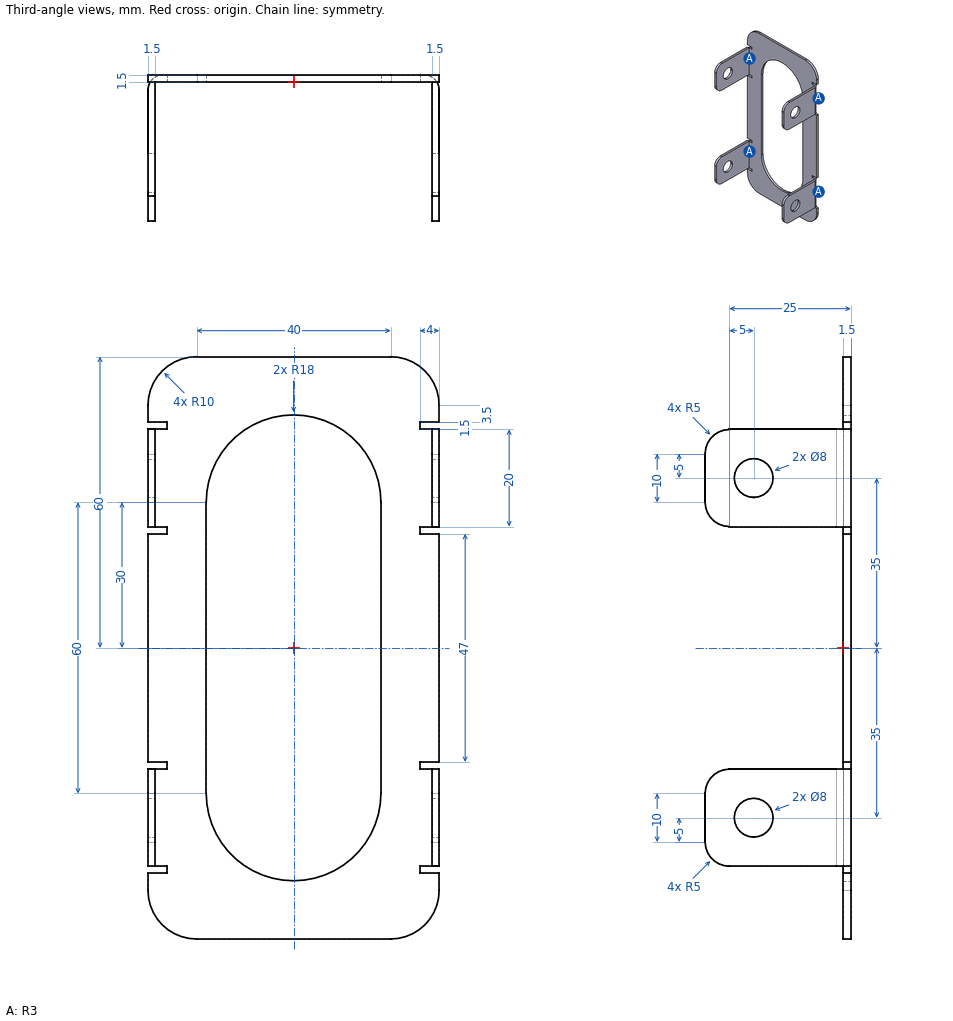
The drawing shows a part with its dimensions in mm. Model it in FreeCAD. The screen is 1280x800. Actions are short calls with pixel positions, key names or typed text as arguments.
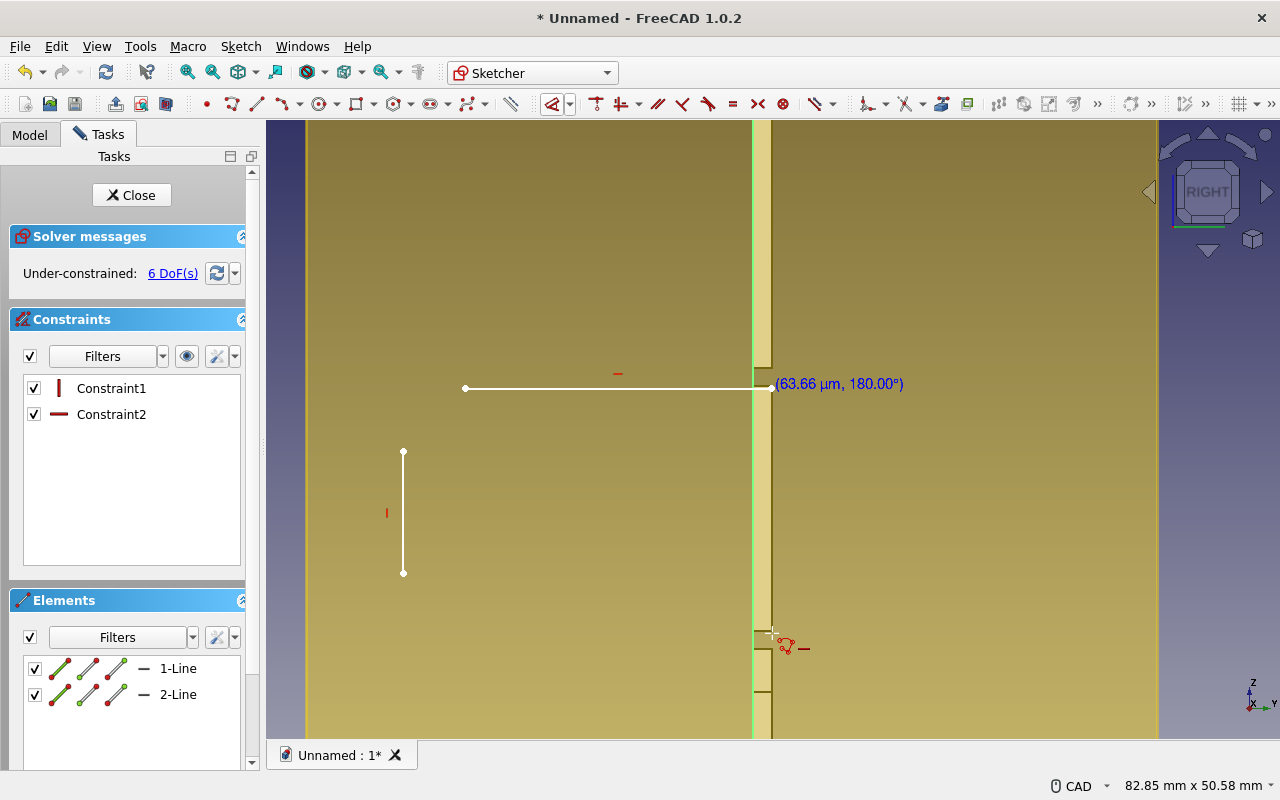
click(772, 631)
click(466, 631)
right_click(466, 631)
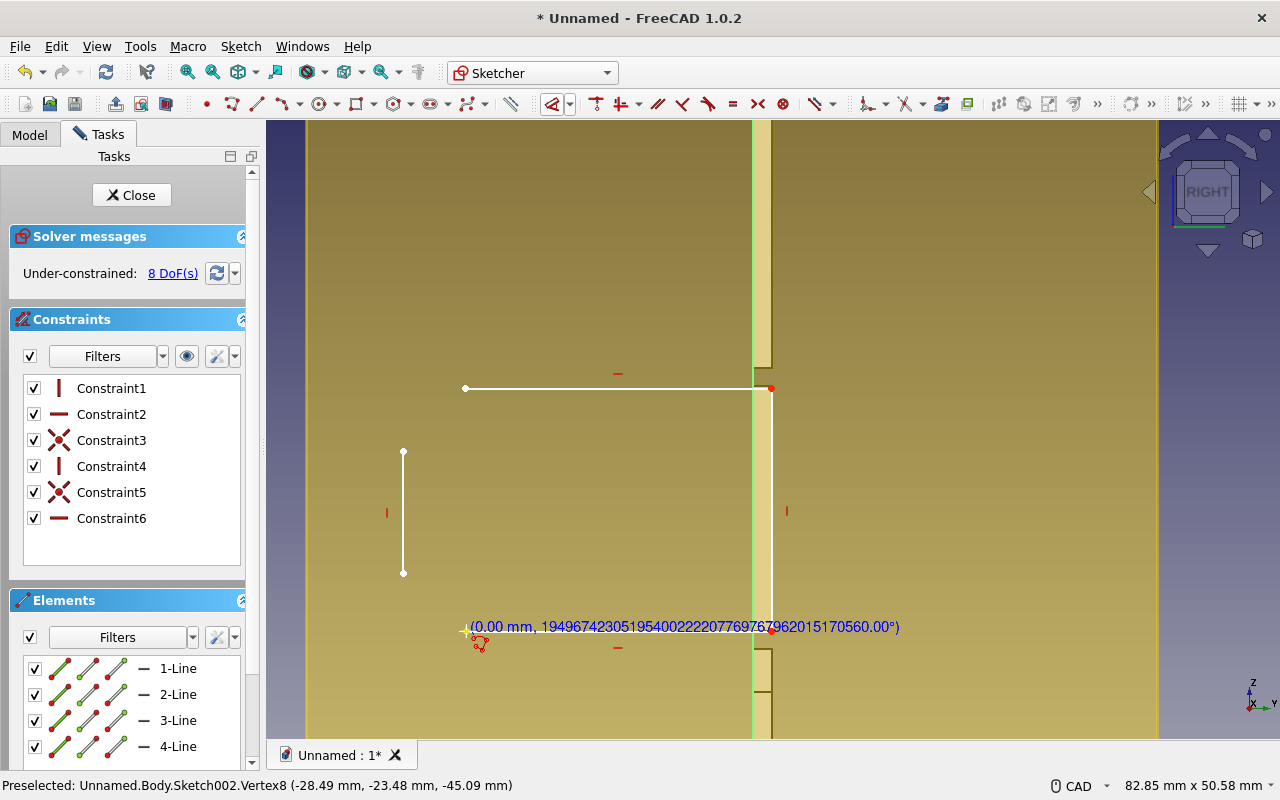
click(282, 104)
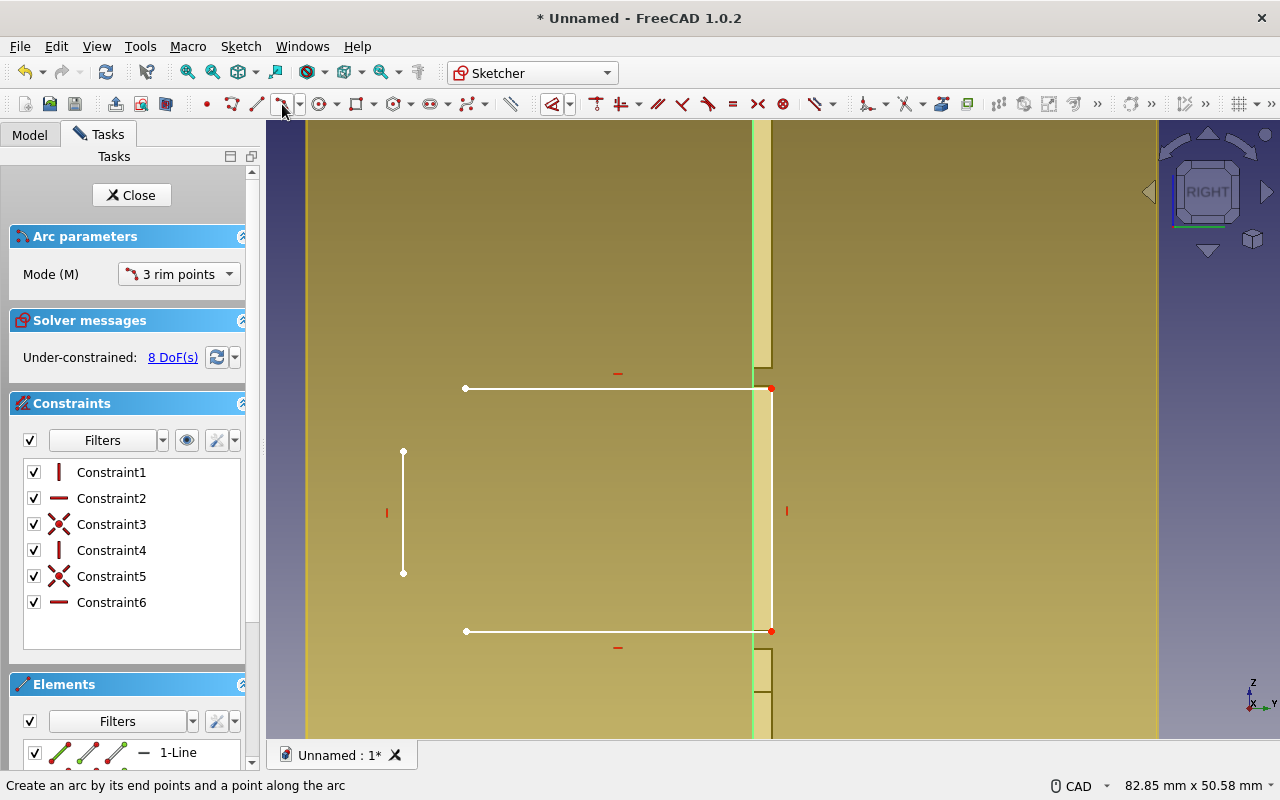
click(403, 451)
click(466, 389)
click(422, 404)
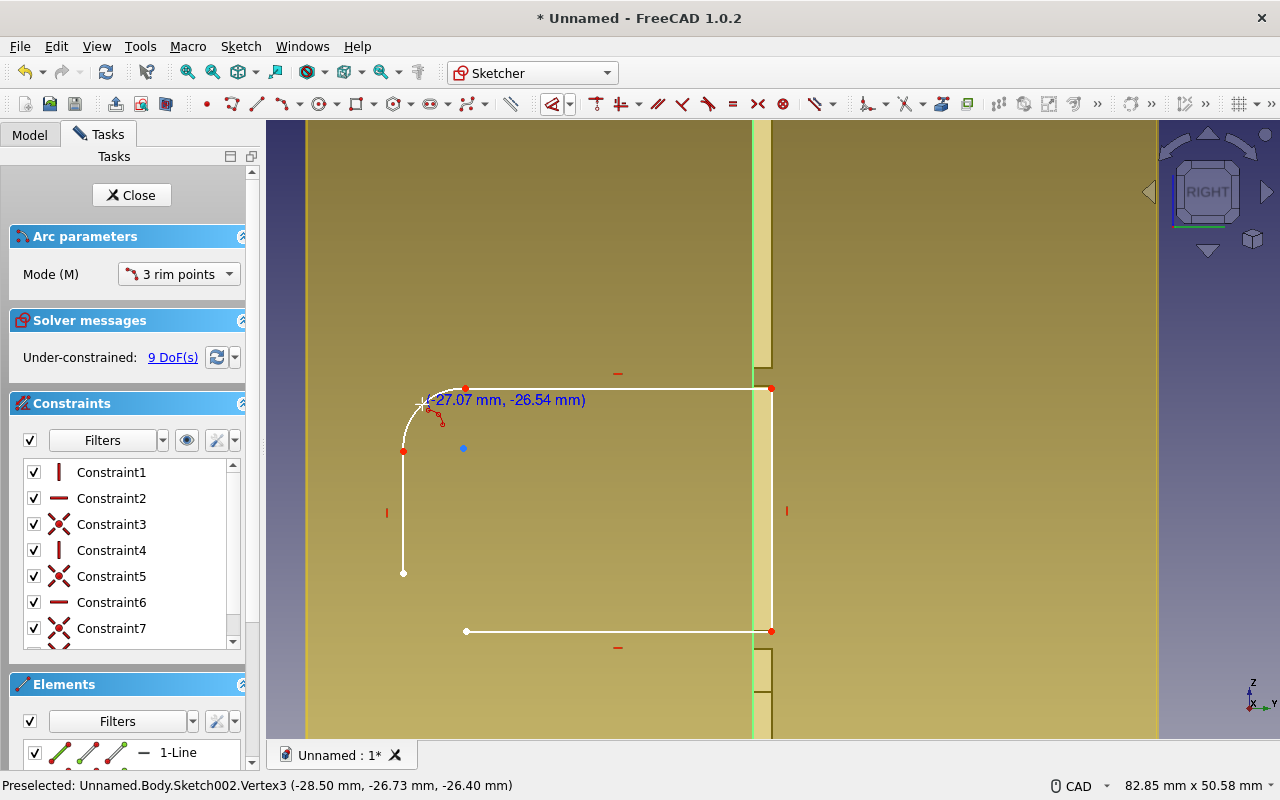
click(466, 632)
click(403, 573)
click(422, 613)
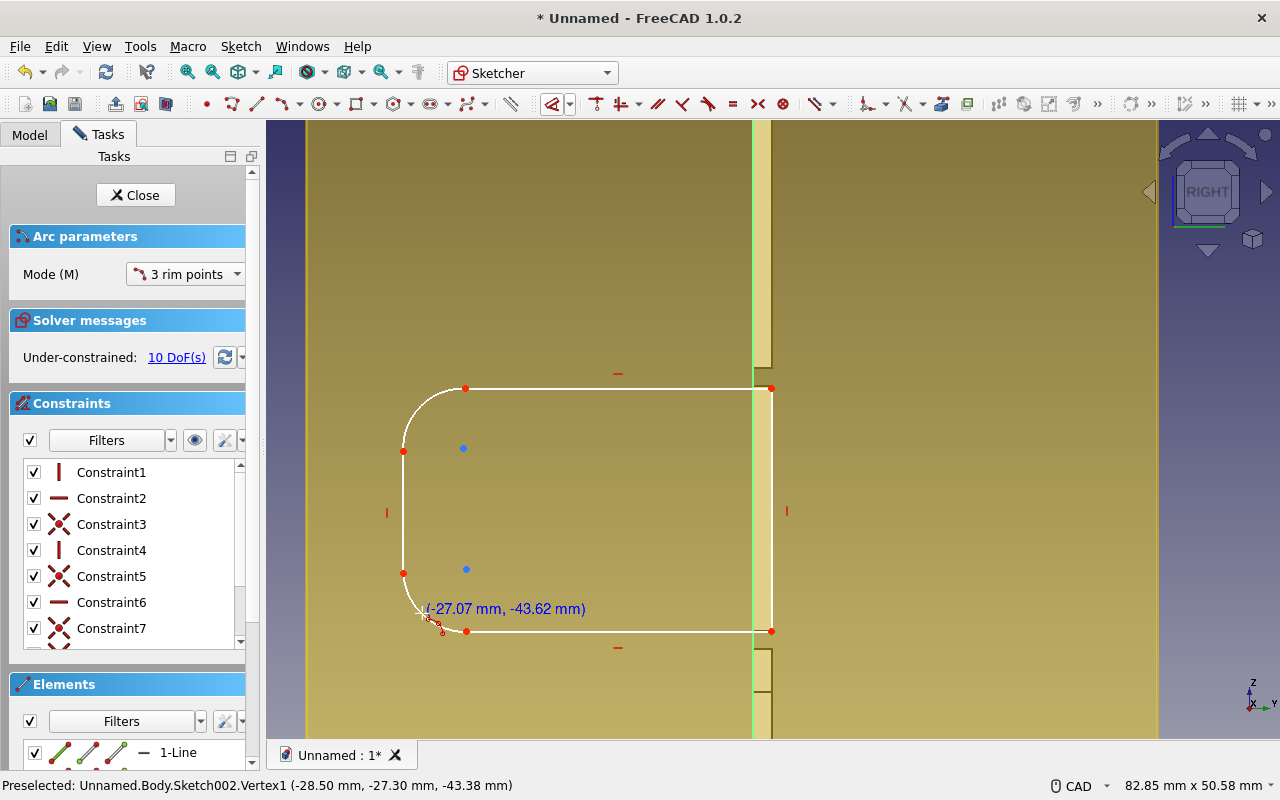
key(g)
key(l)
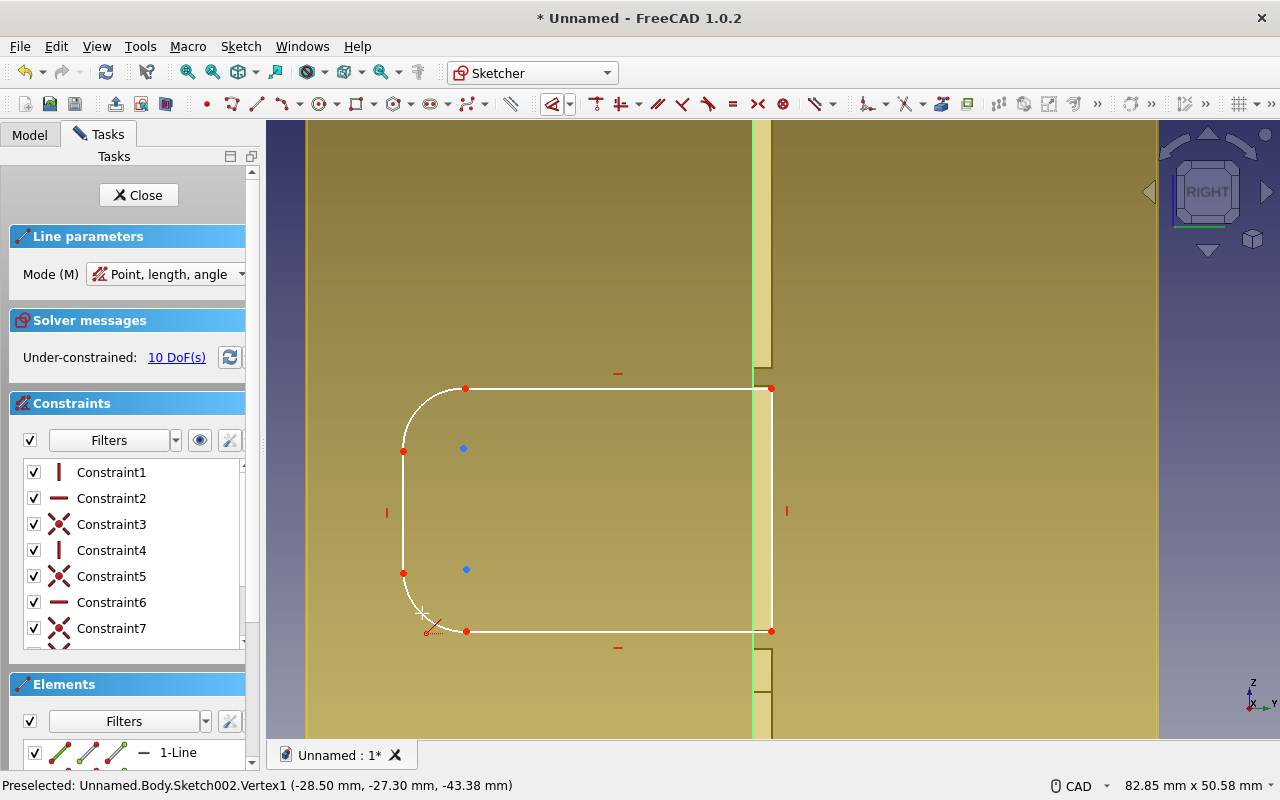
scroll(772, 633, down, 5)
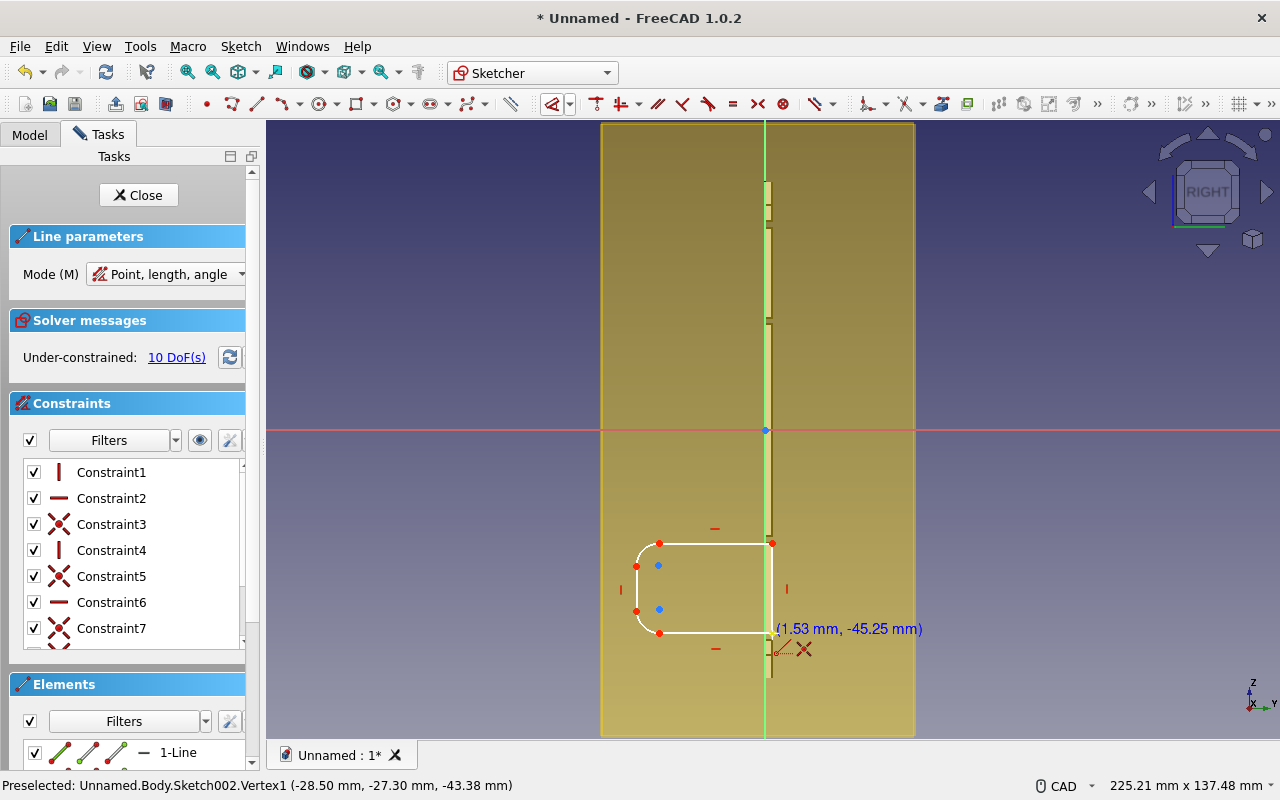
click(637, 295)
click(637, 250)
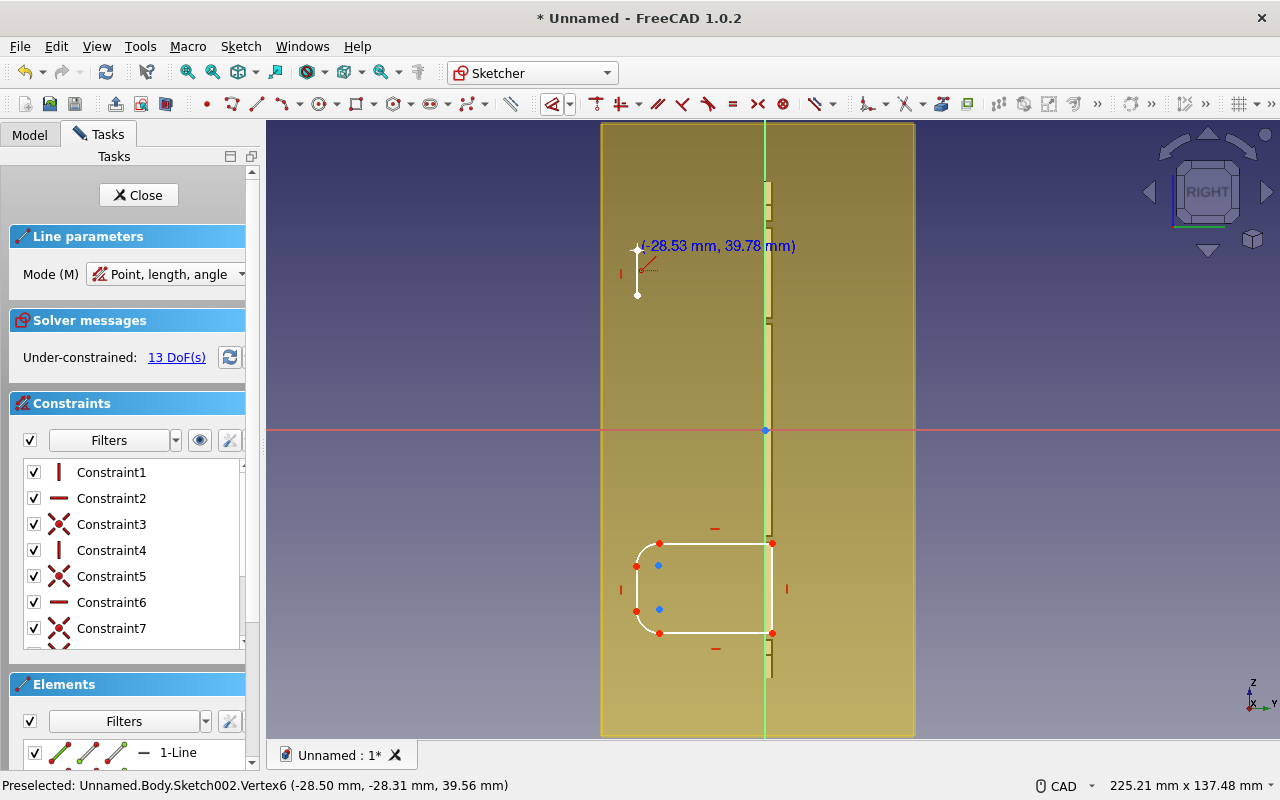
click(232, 104)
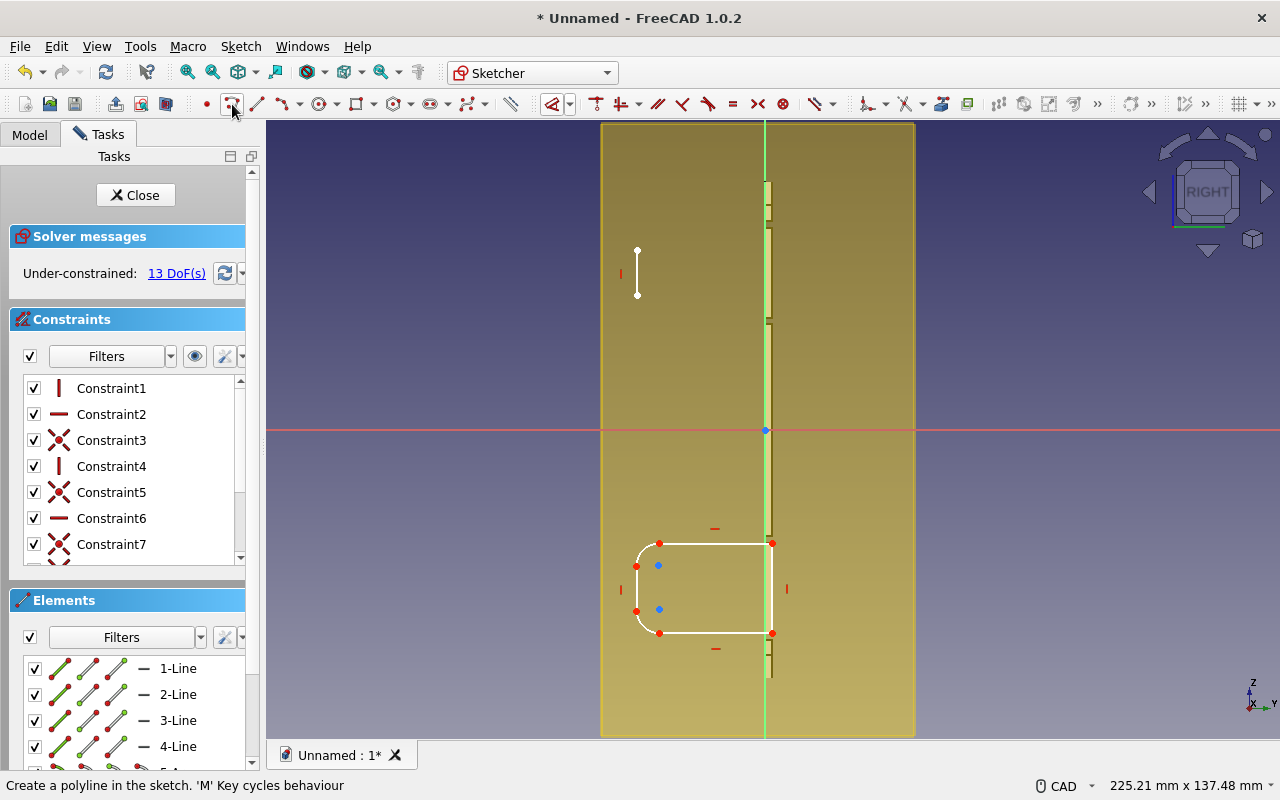
click(660, 228)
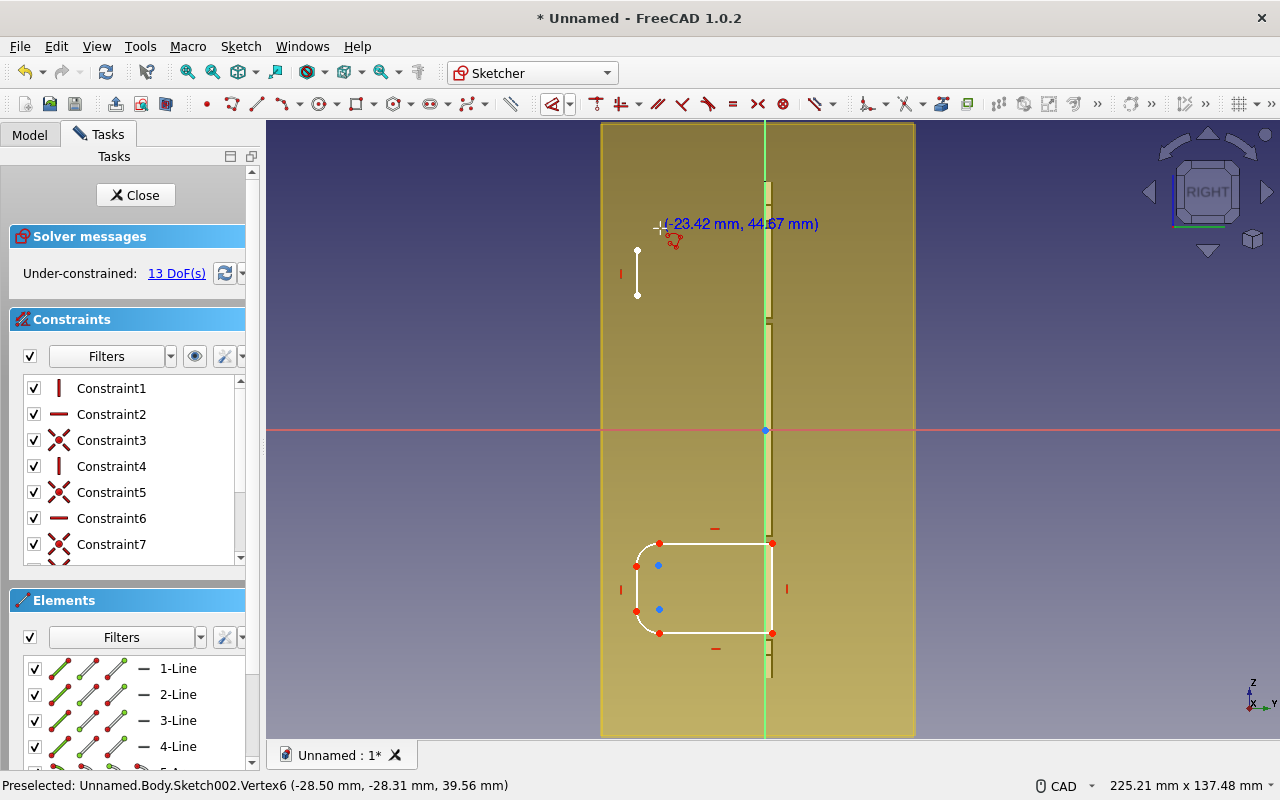
scroll(772, 228, up, 5)